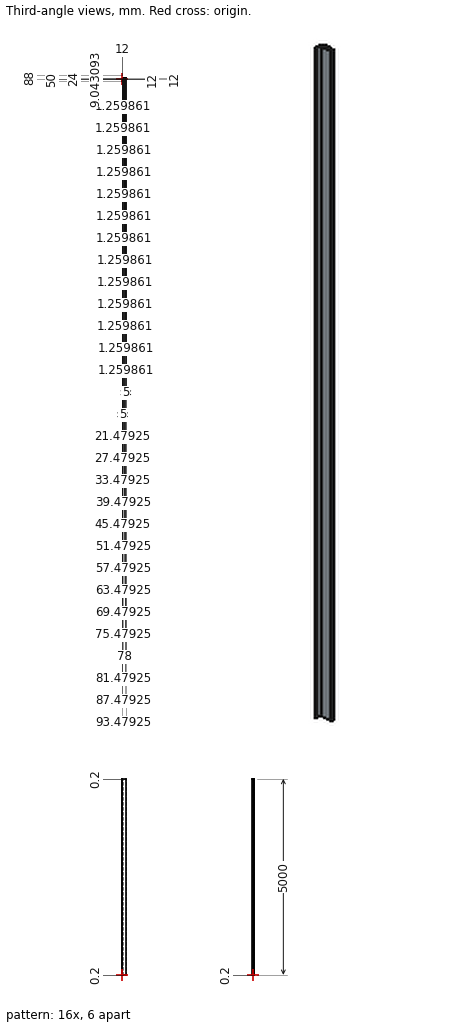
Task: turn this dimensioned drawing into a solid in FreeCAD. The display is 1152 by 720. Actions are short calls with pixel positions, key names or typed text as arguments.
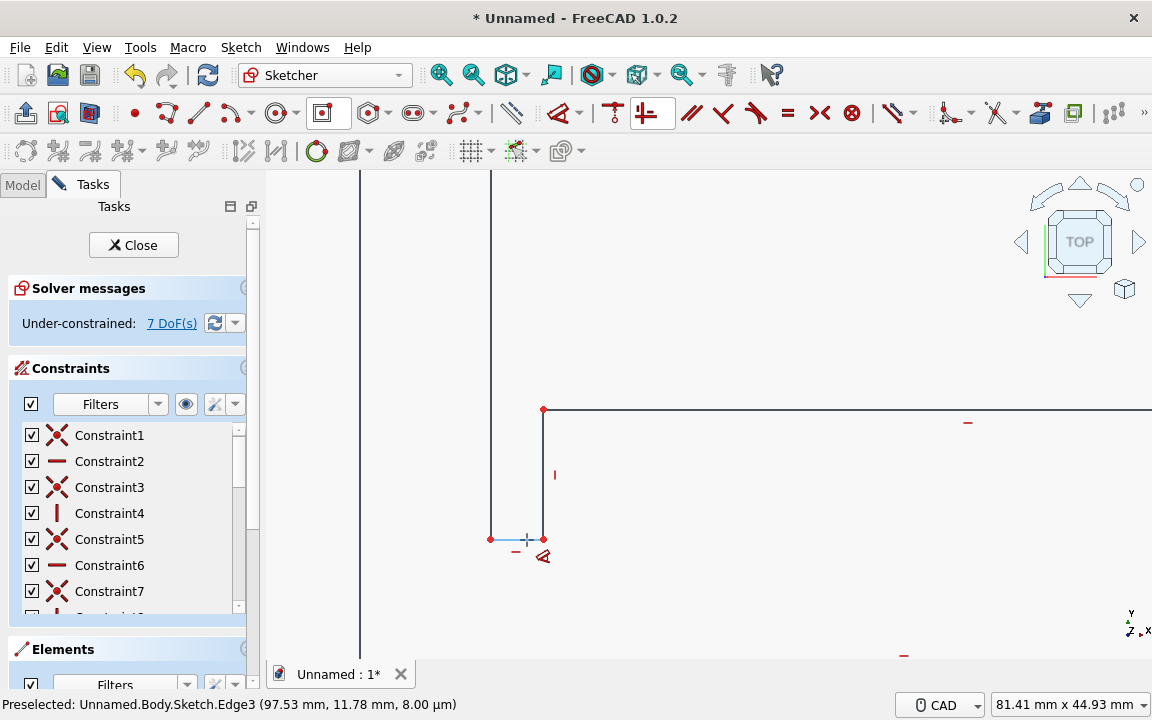
click(527, 540)
click(517, 574)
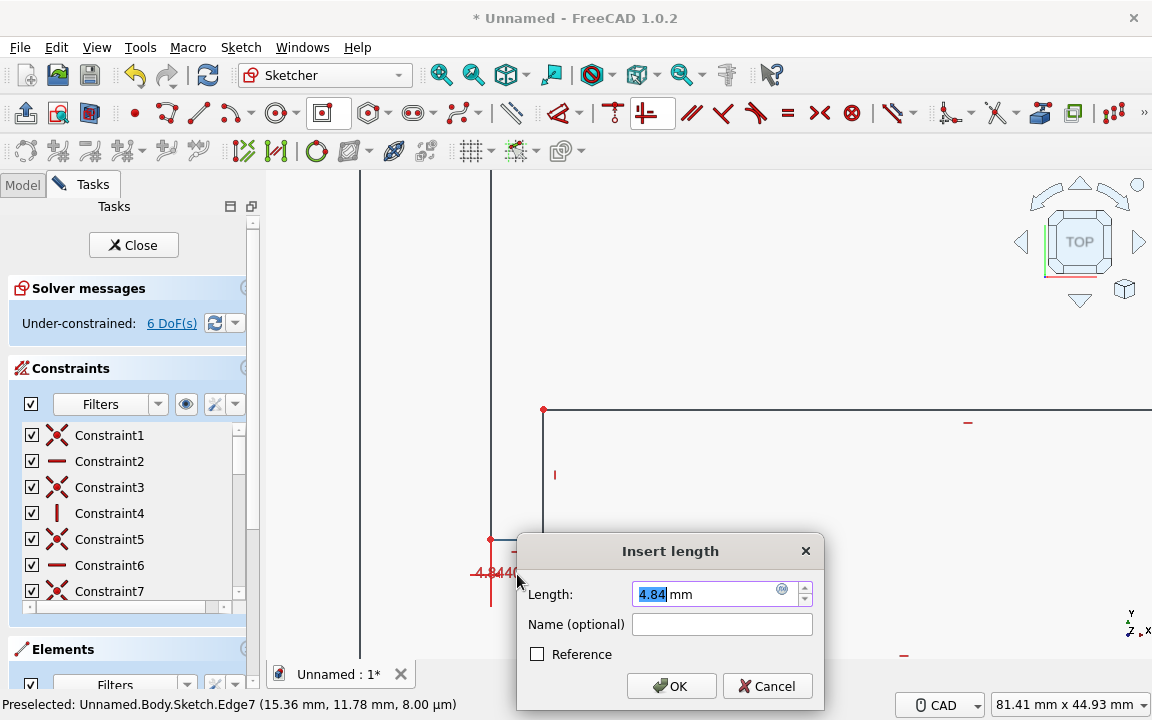
text(5)
key(Return)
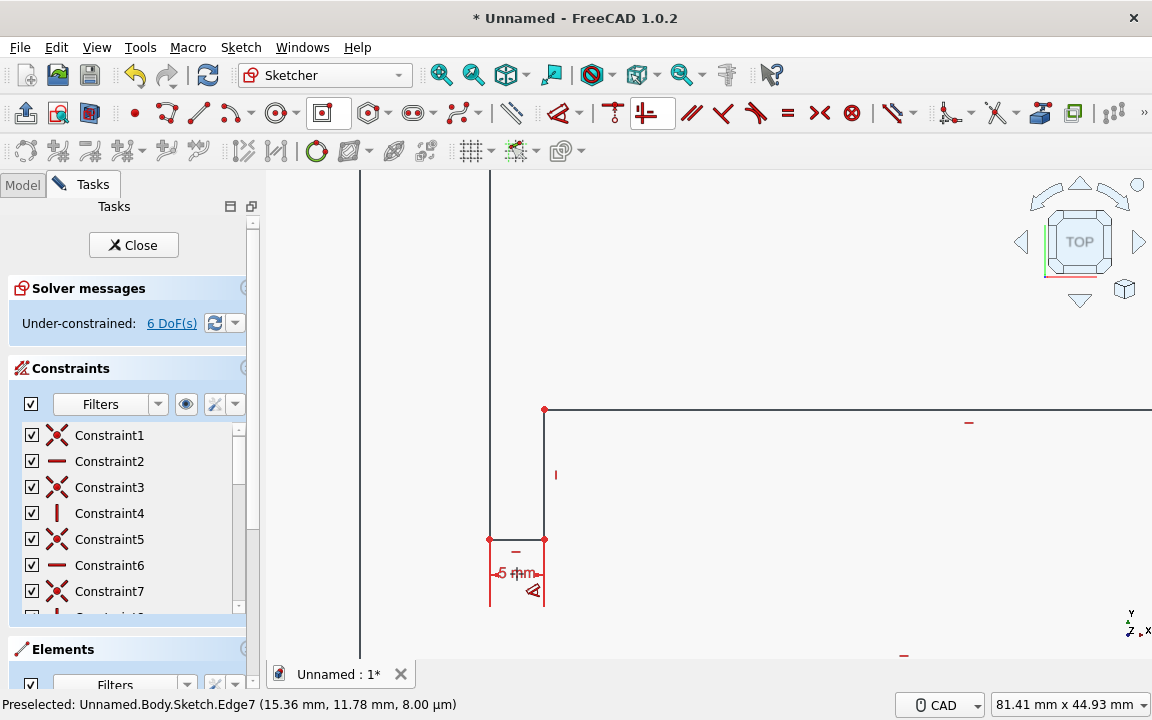
scroll(527, 540, down, 6)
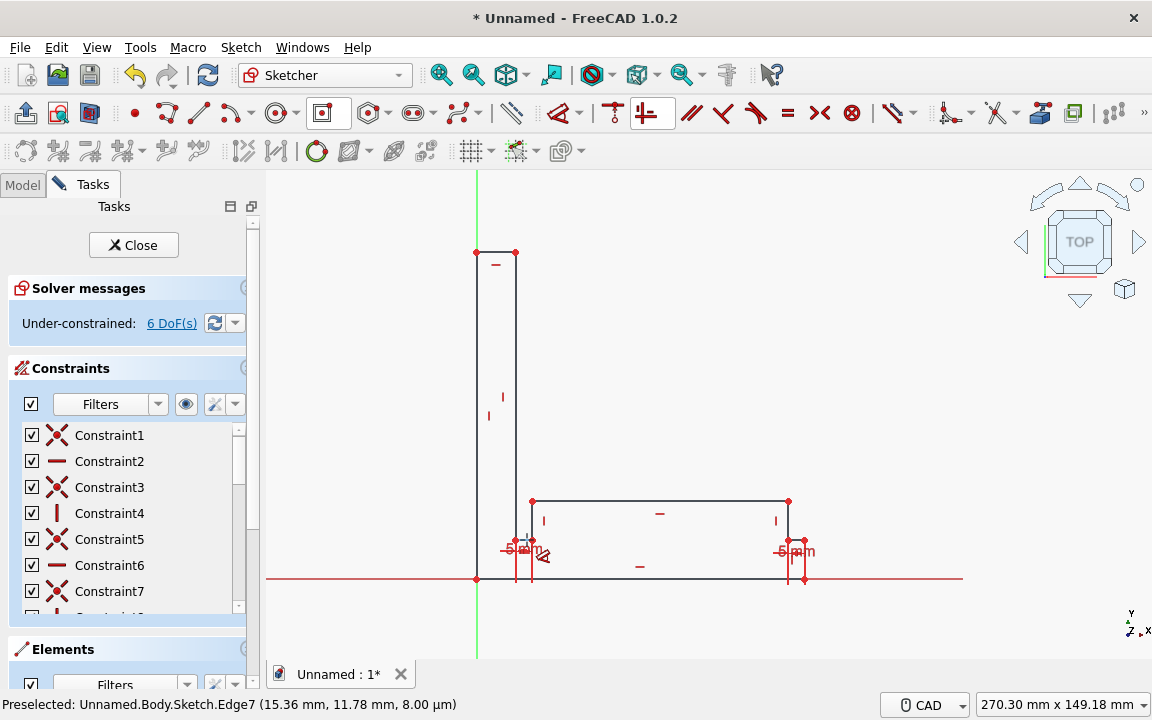
click(805, 567)
click(887, 560)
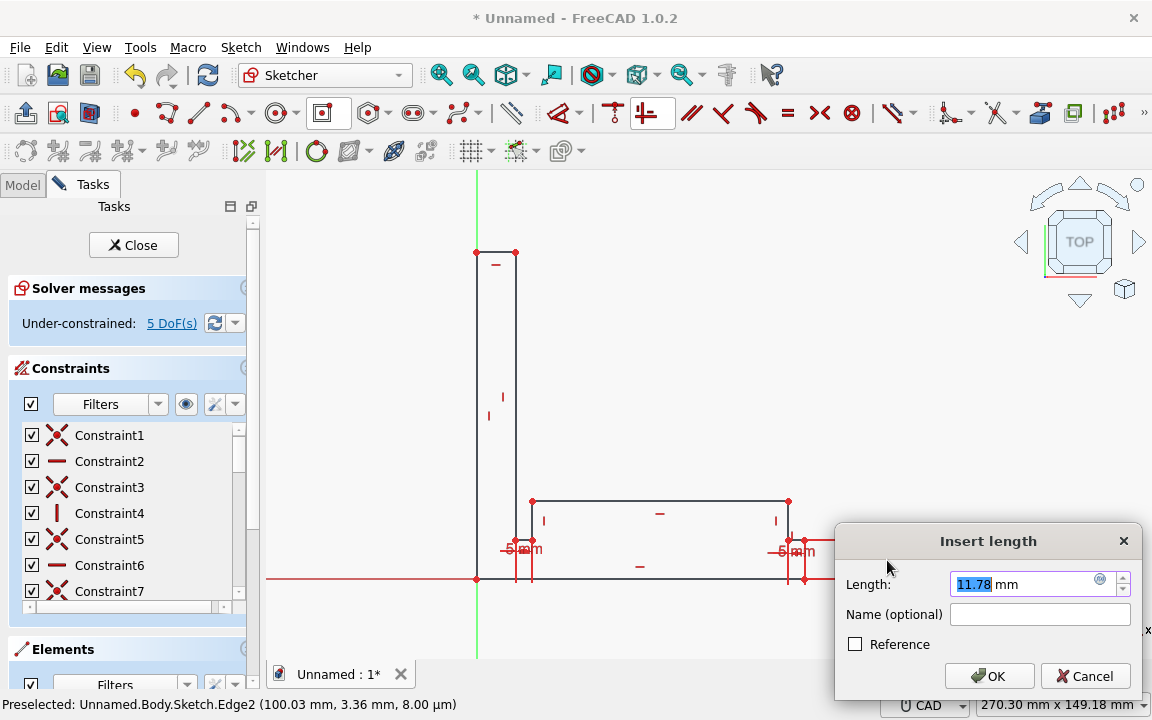
text(12)
key(Return)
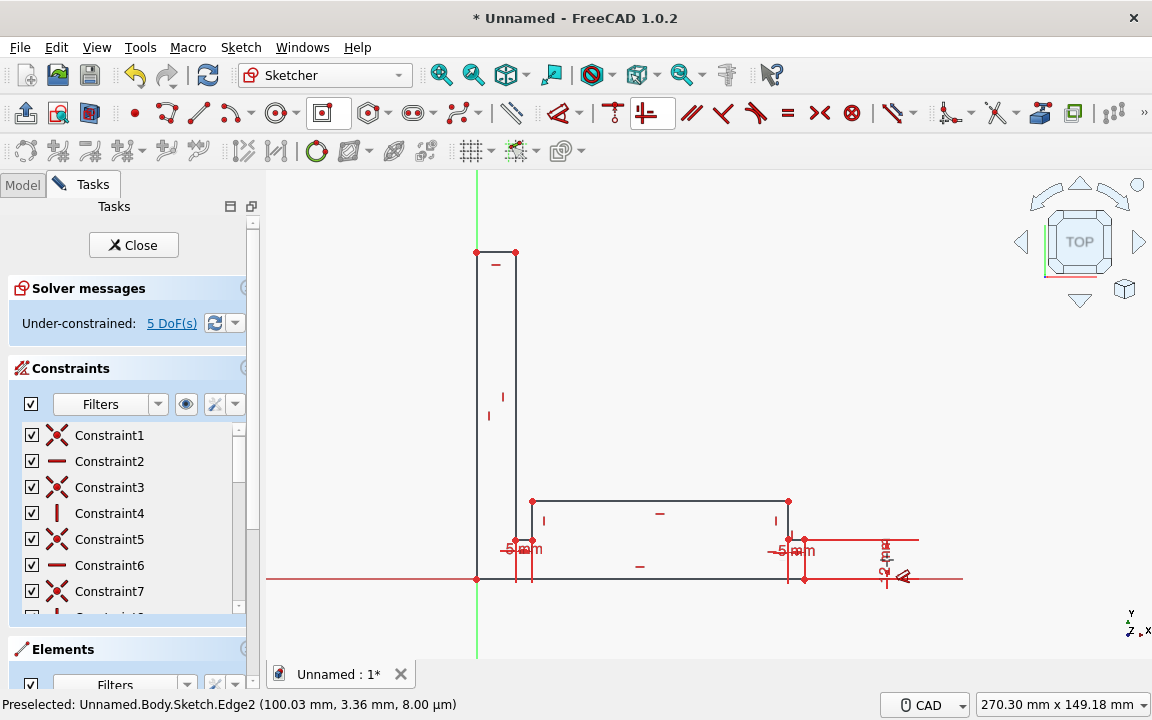
click(788, 528)
click(822, 520)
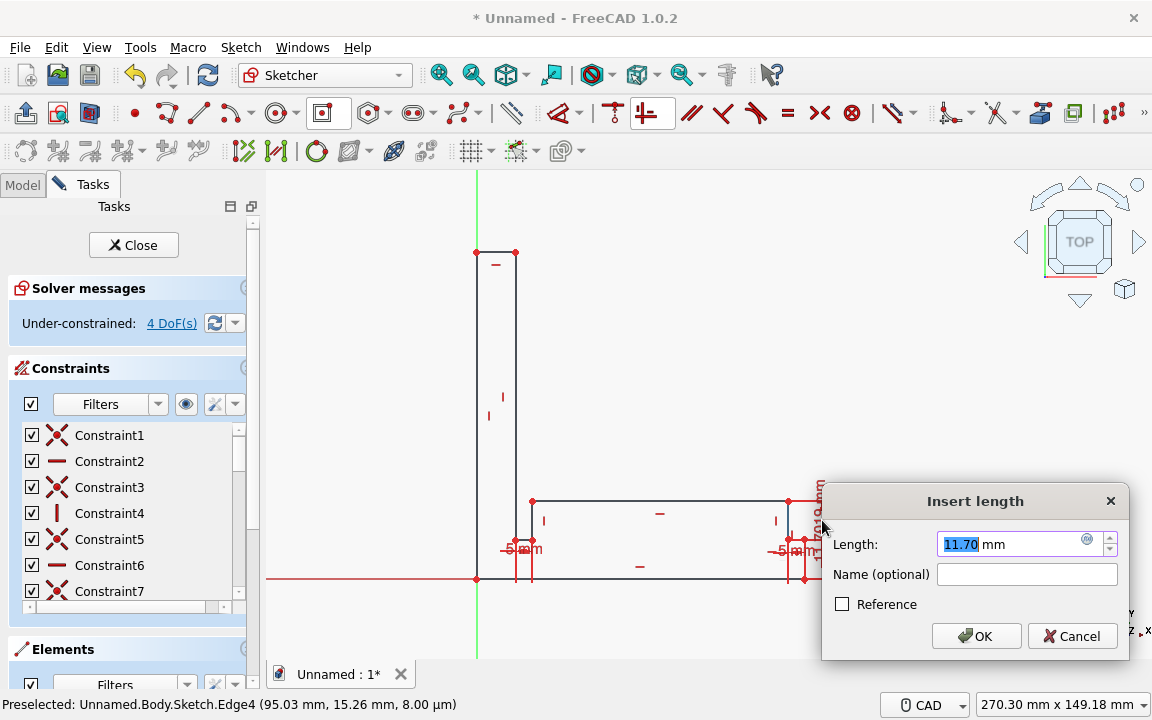
text(12)
key(Return)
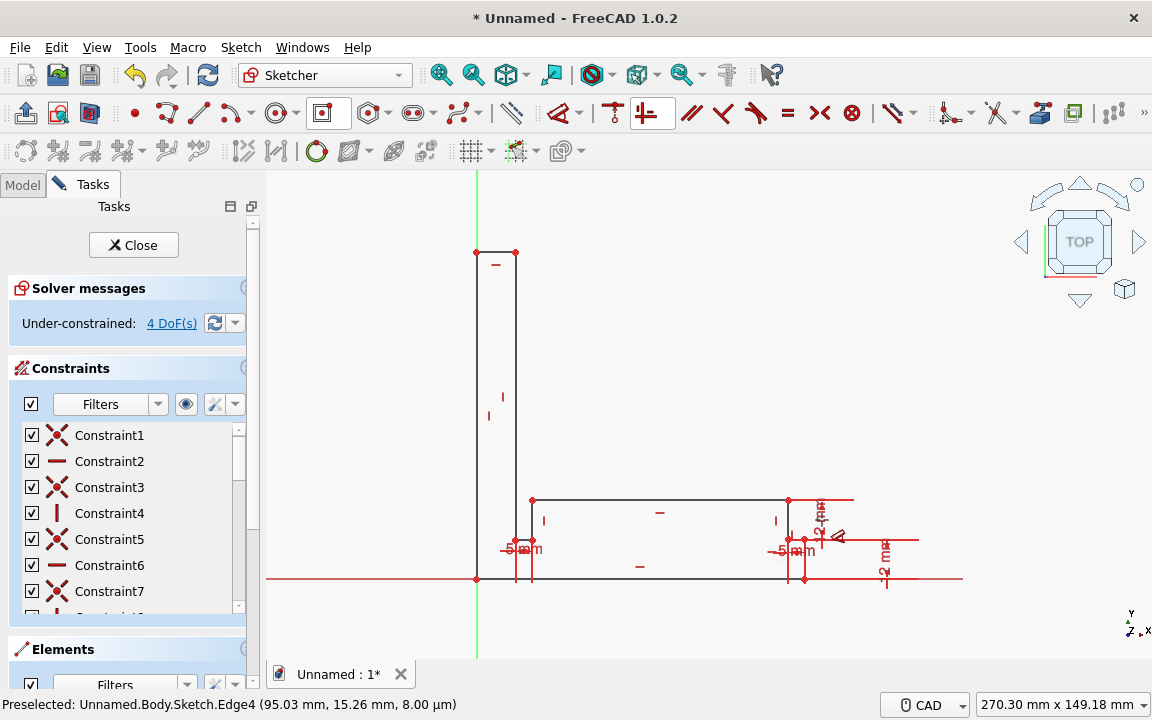
click(712, 500)
click(660, 534)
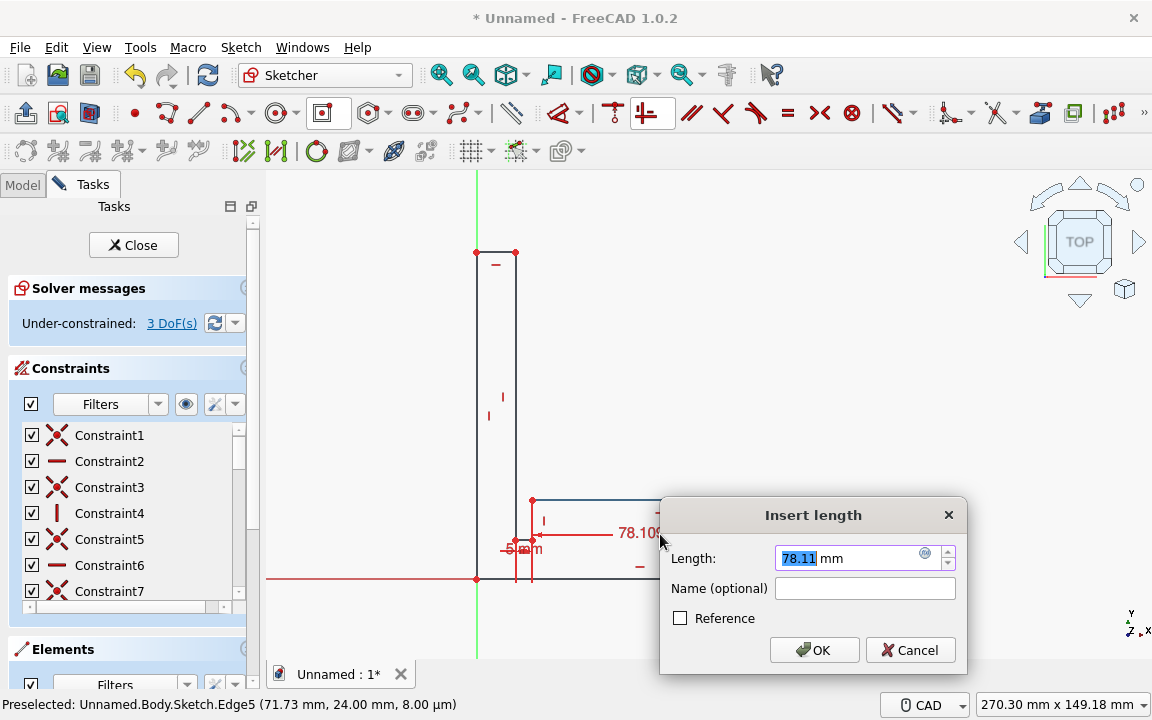
text(78)
key(Return)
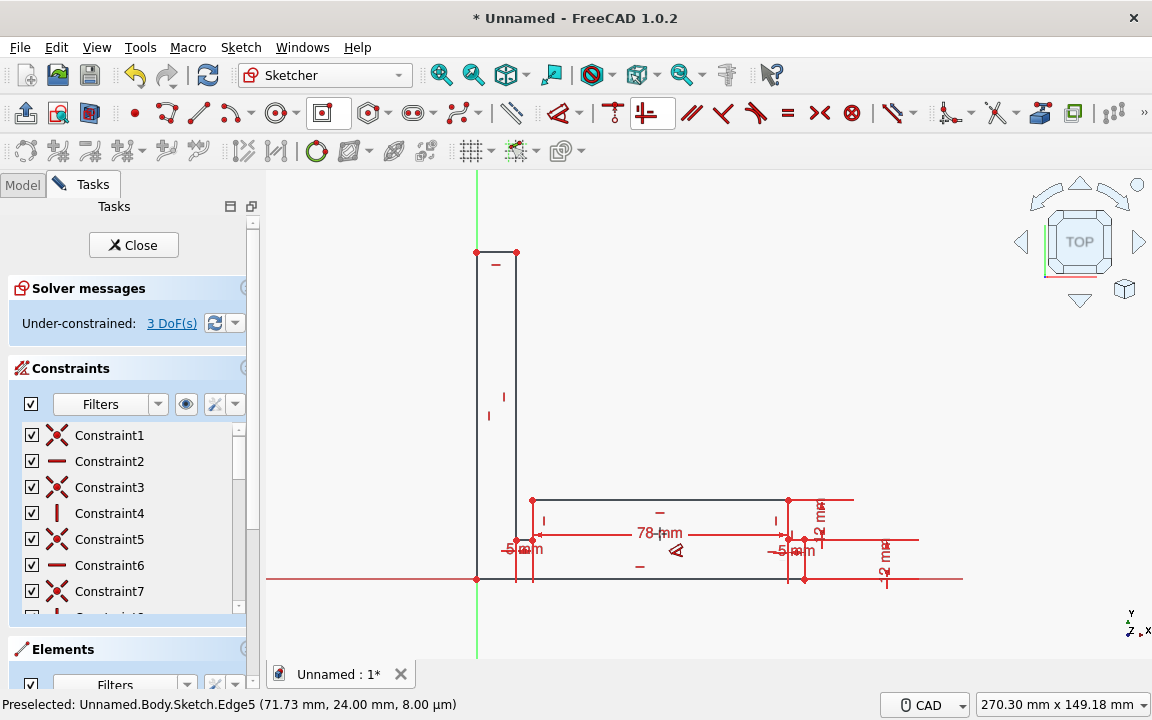
click(533, 512)
click(499, 520)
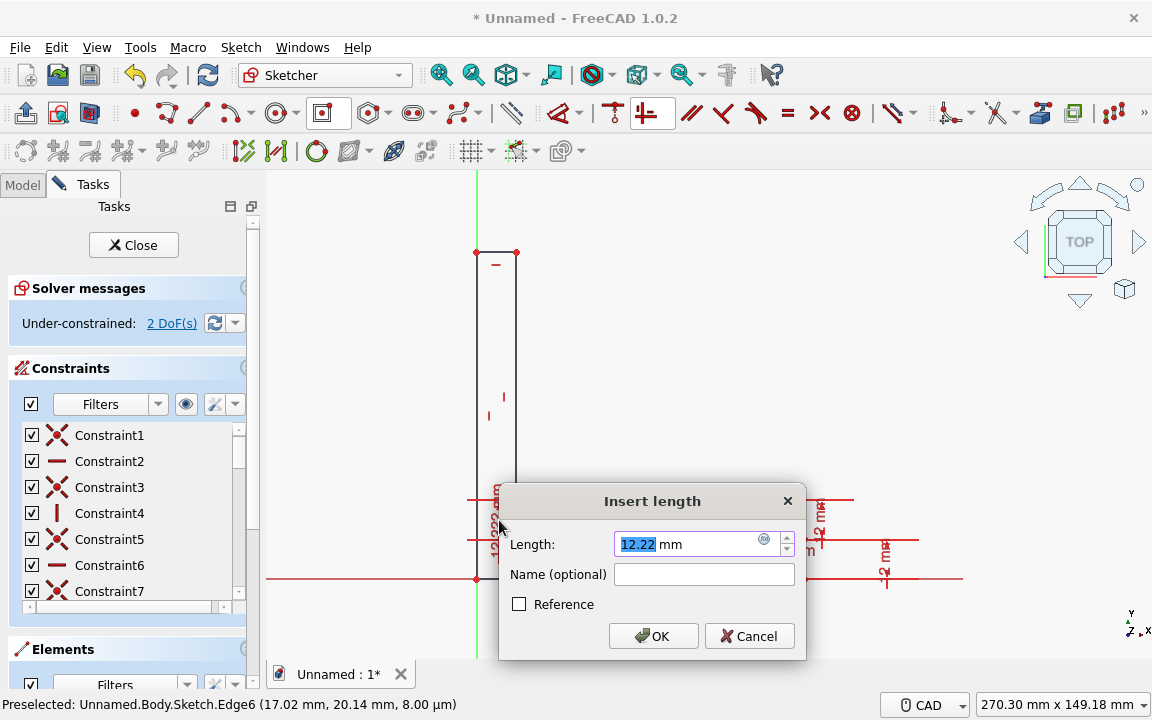
text(12)
key(Return)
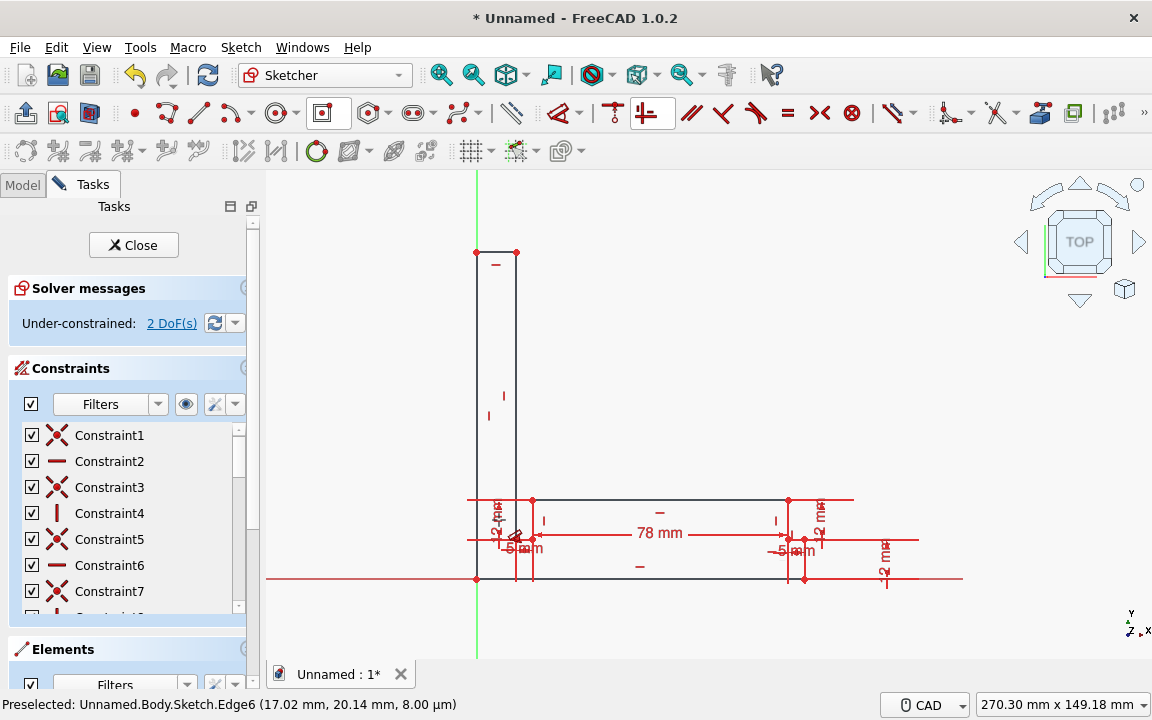
click(516, 453)
click(550, 396)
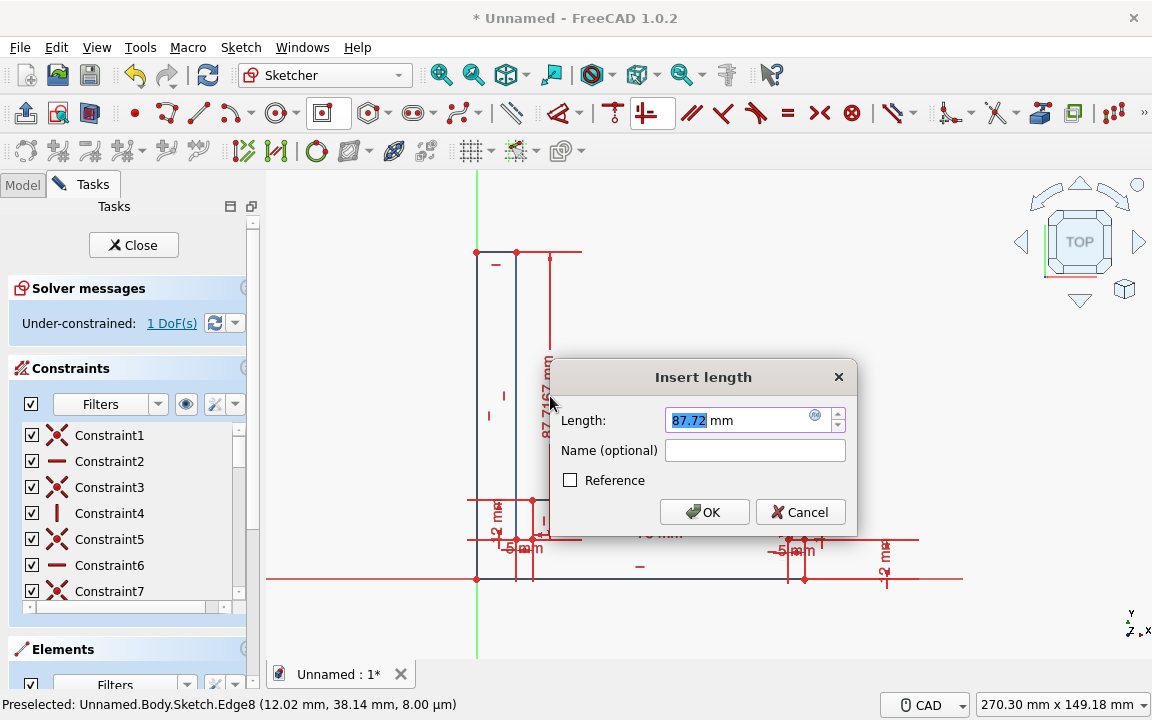
text(88)
key(Return)